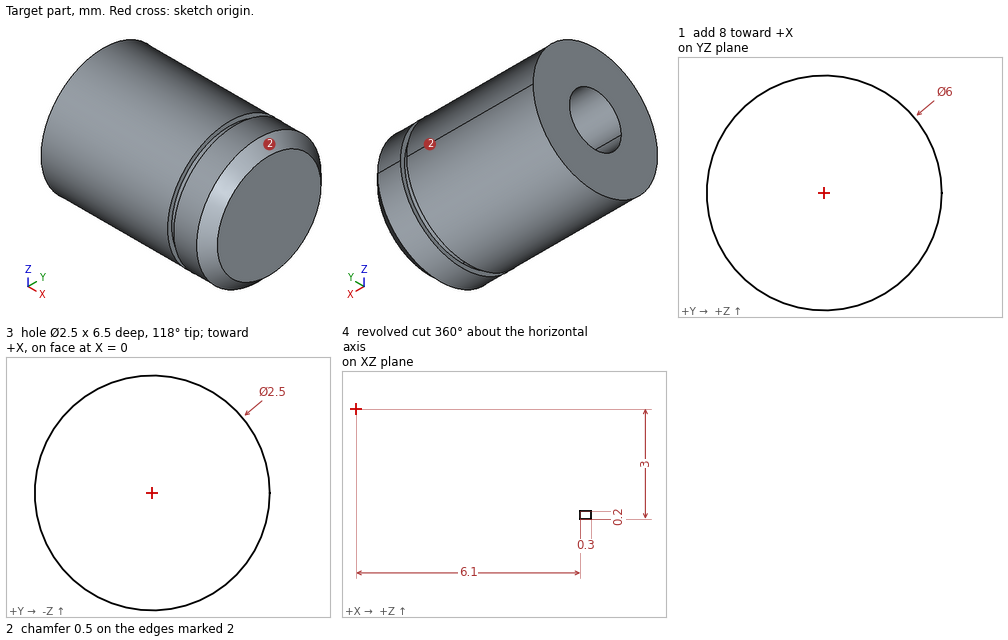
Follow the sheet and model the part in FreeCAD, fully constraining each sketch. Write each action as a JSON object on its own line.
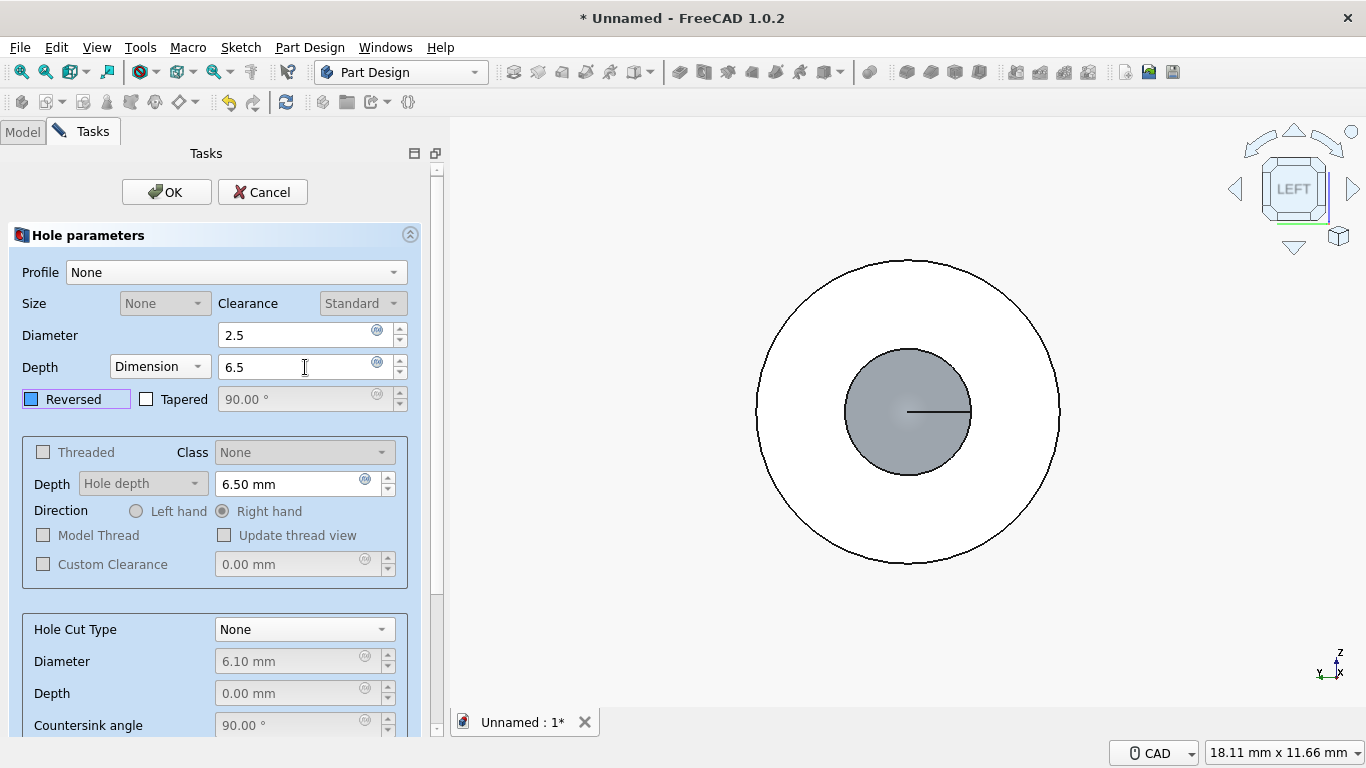
{"action": "left_click", "coordinate": [167, 192]}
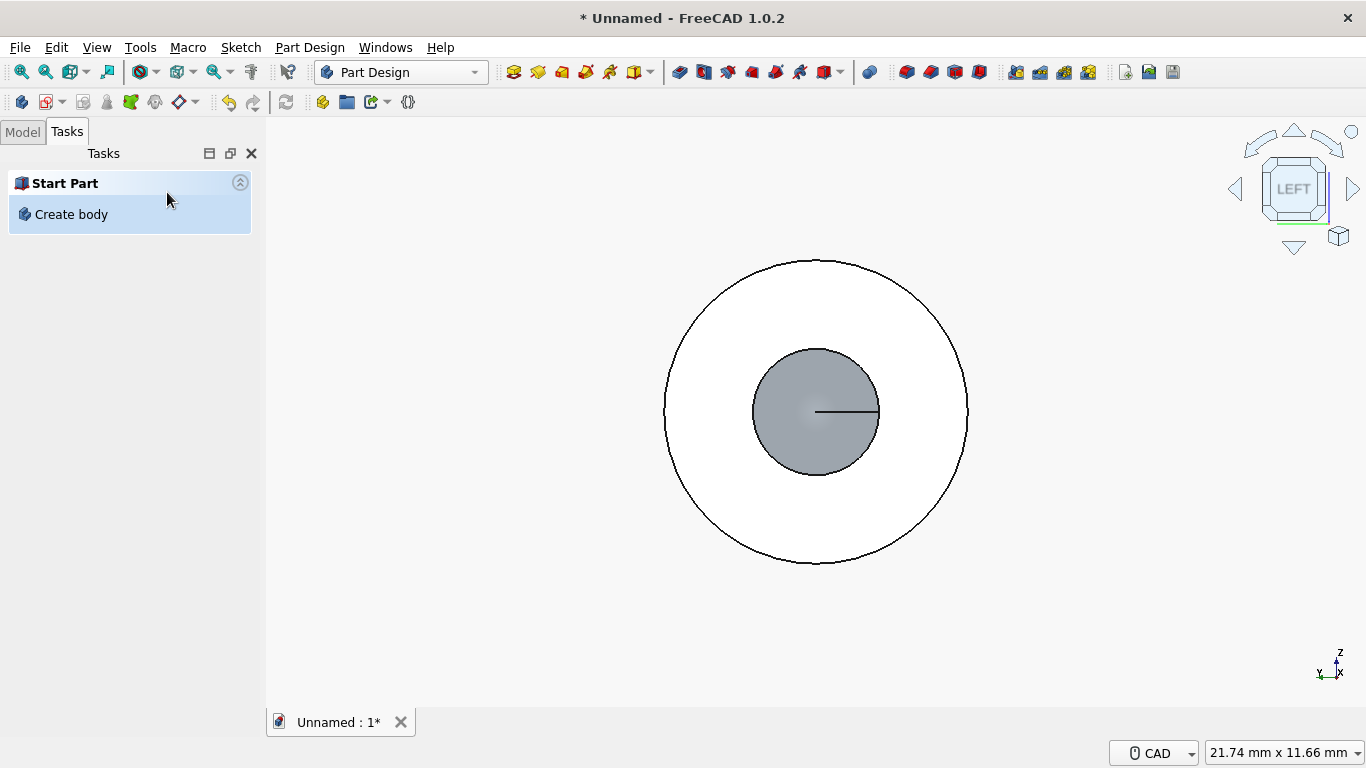
{"action": "left_click", "coordinate": [46, 102]}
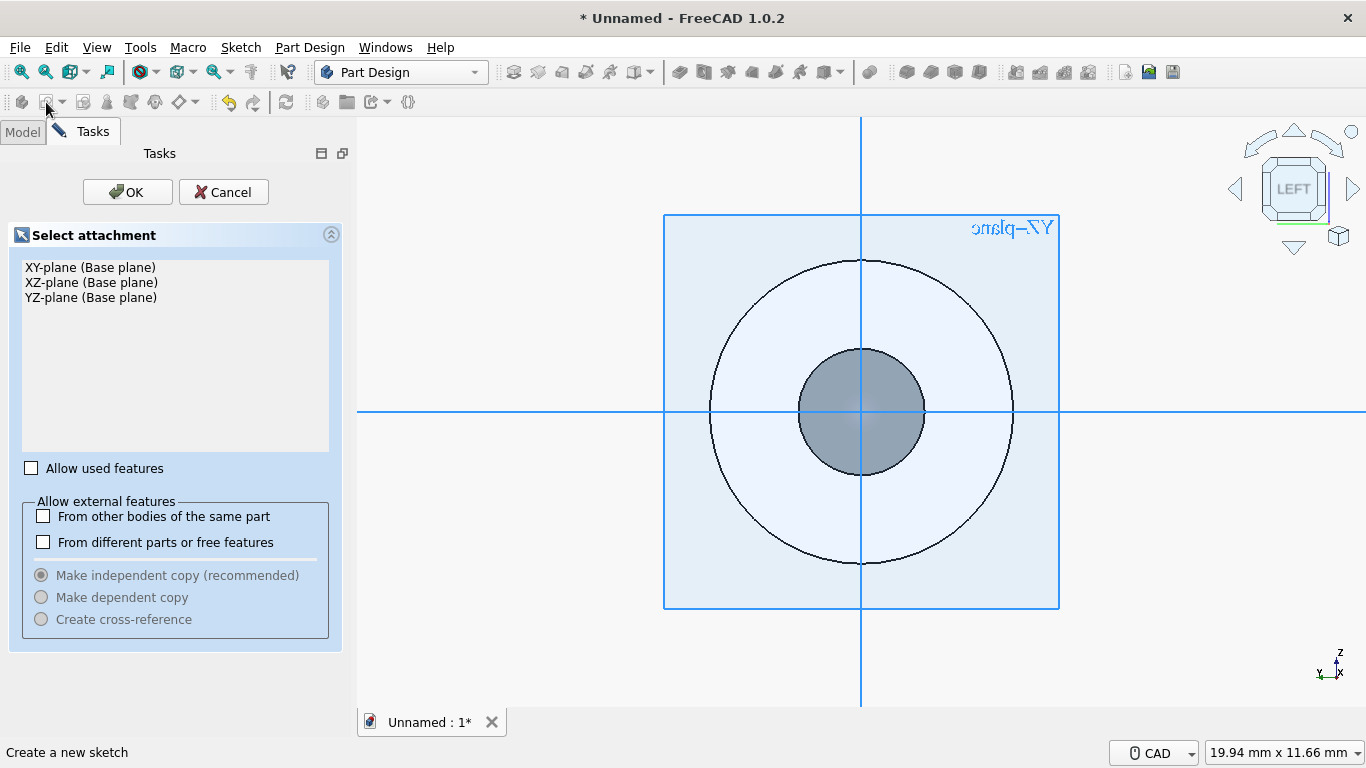
{"action": "left_click", "coordinate": [82, 282]}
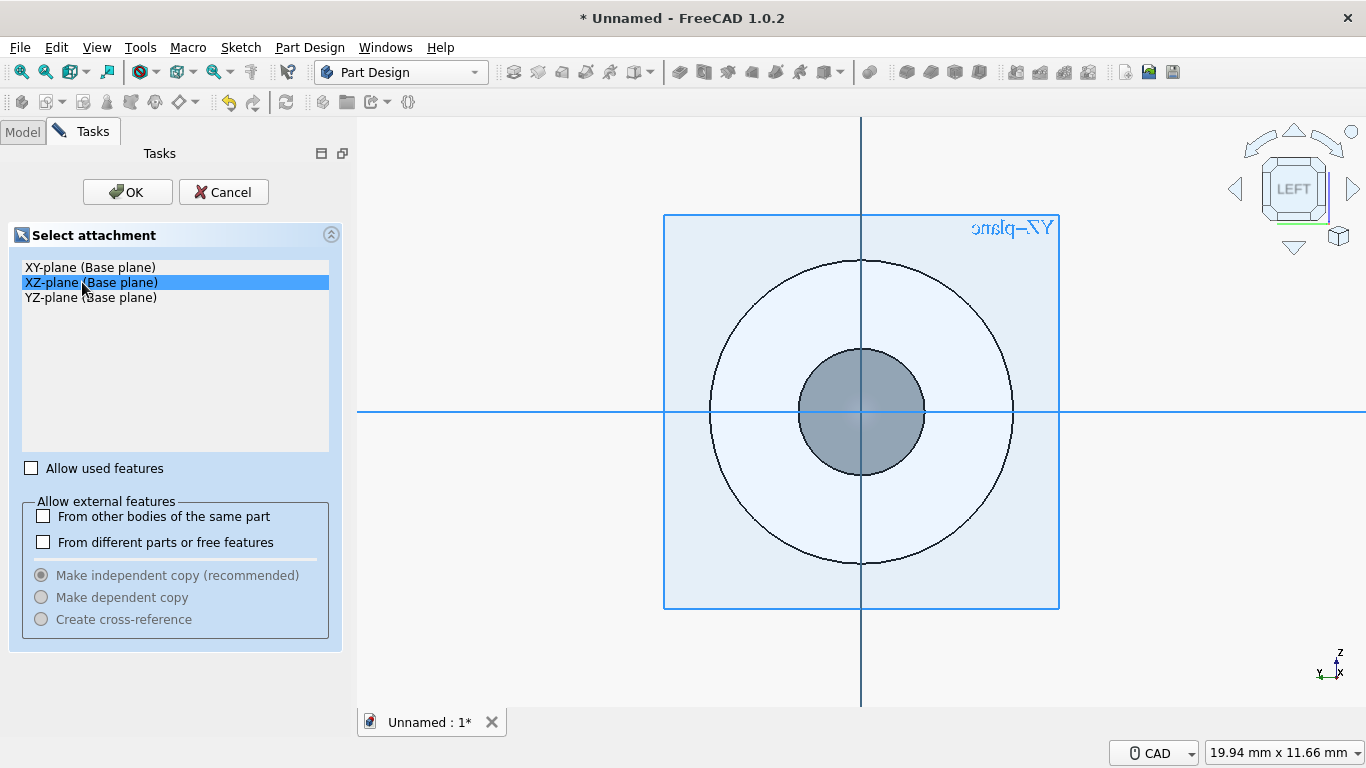
{"action": "left_click", "coordinate": [128, 192]}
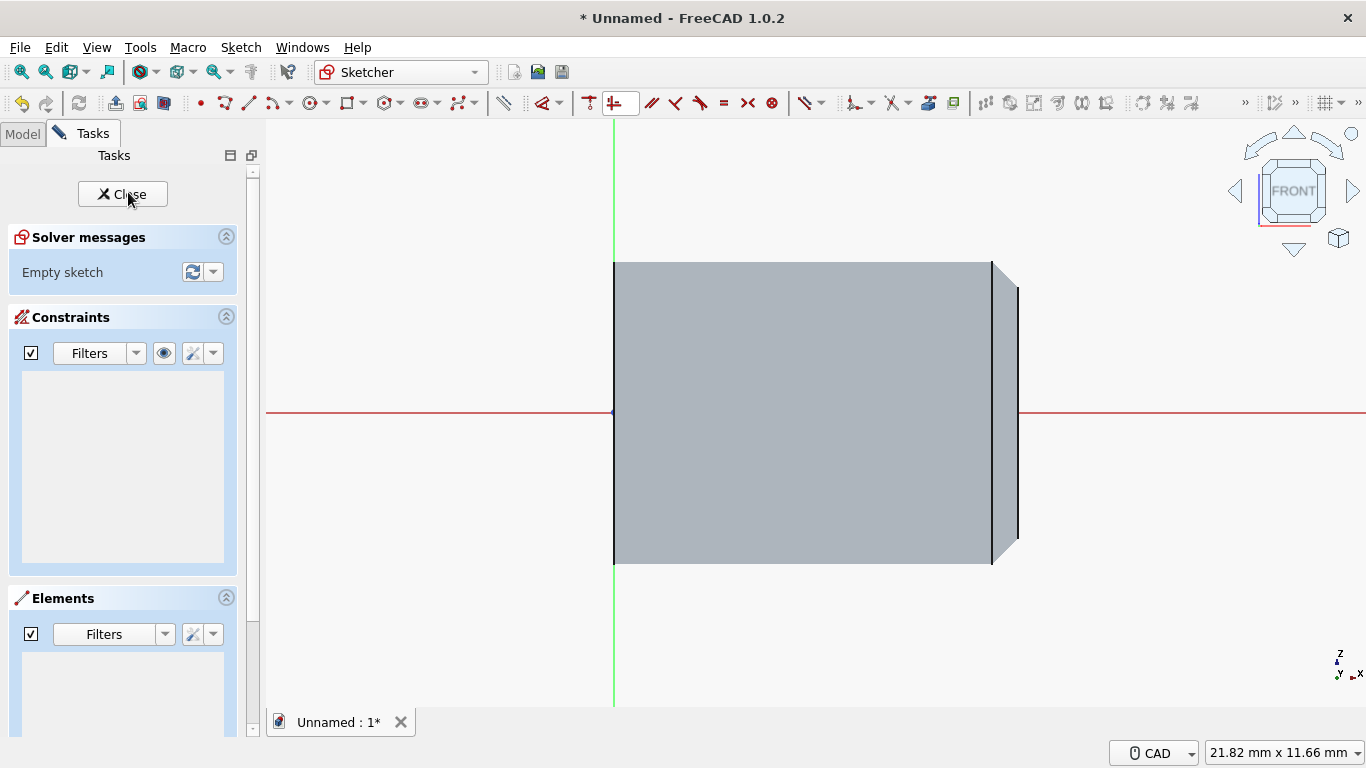
{"action": "left_click", "coordinate": [164, 104]}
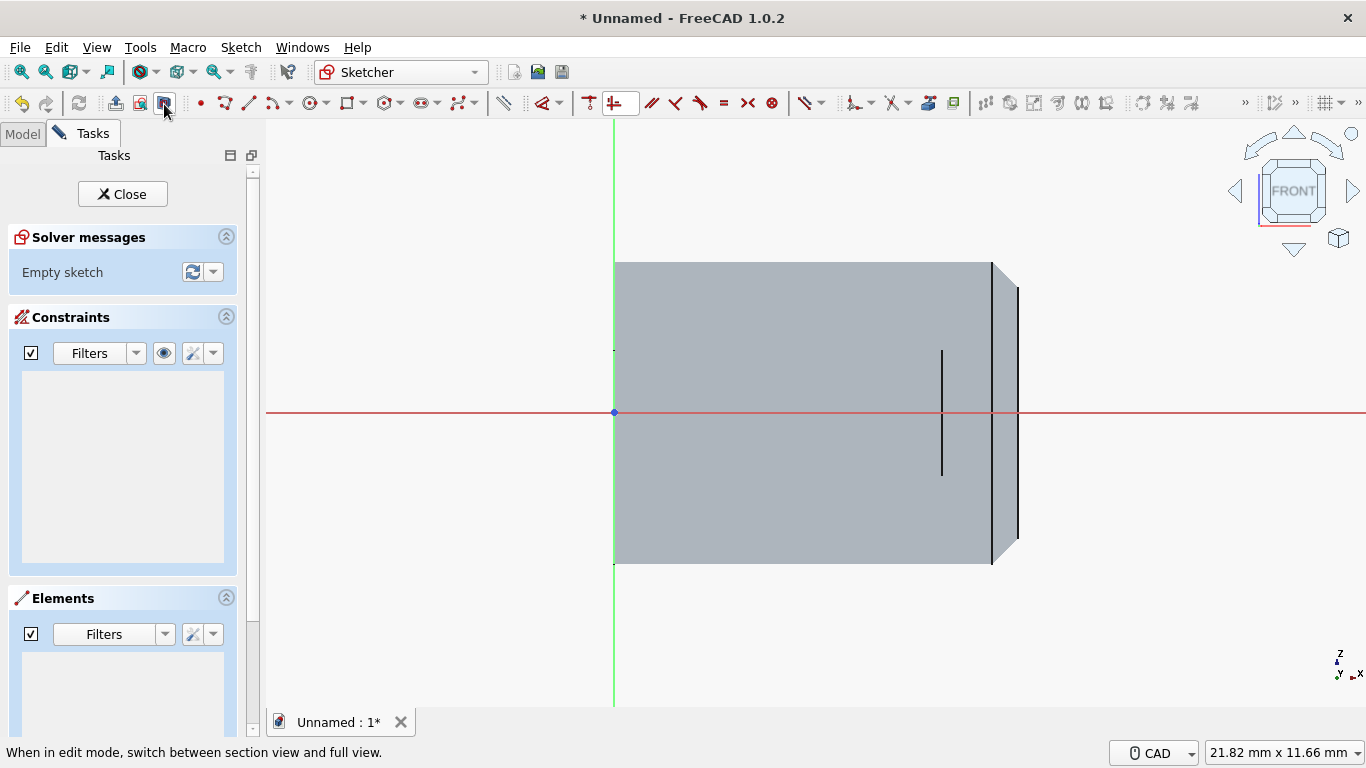
{"action": "scroll", "coordinate": [939, 567], "scroll_direction": "up", "scroll_amount": 15}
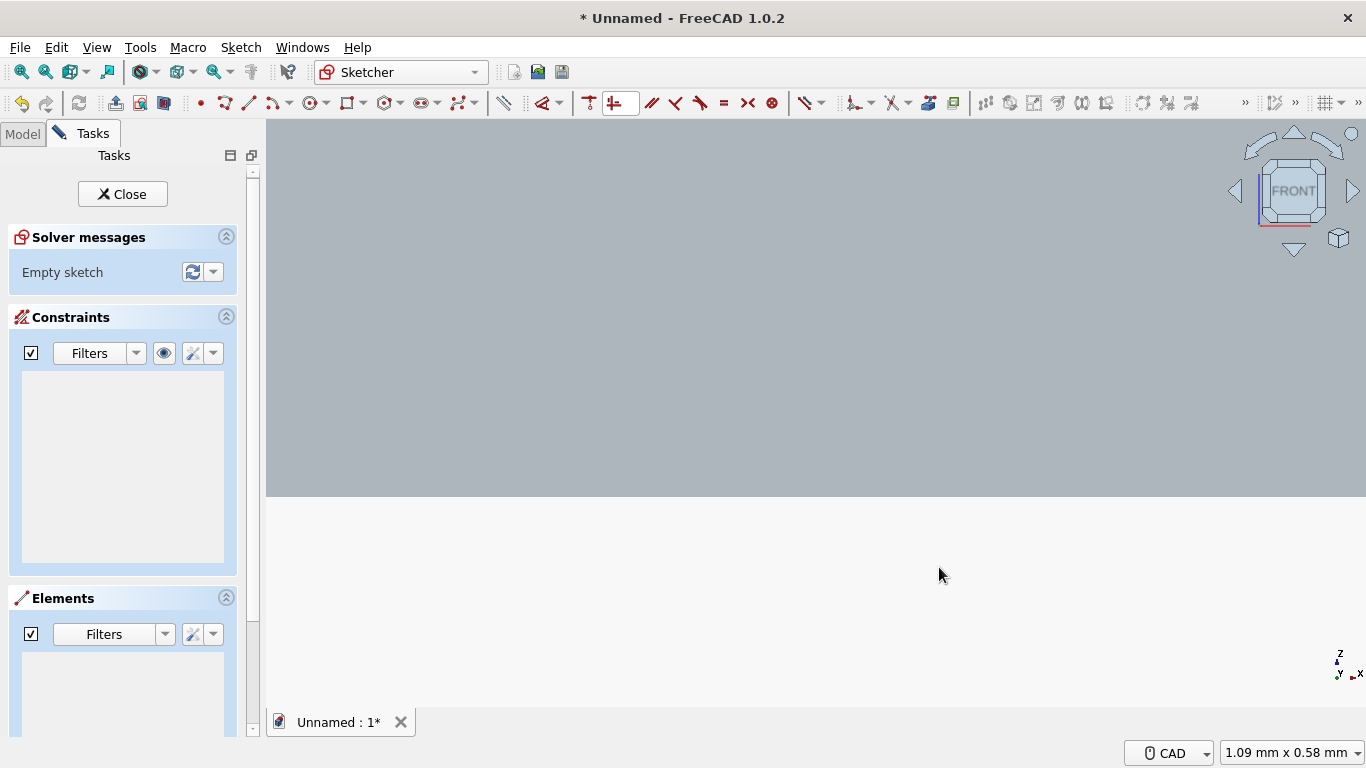
{"action": "scroll", "coordinate": [721, 376], "scroll_direction": "up", "scroll_amount": 3}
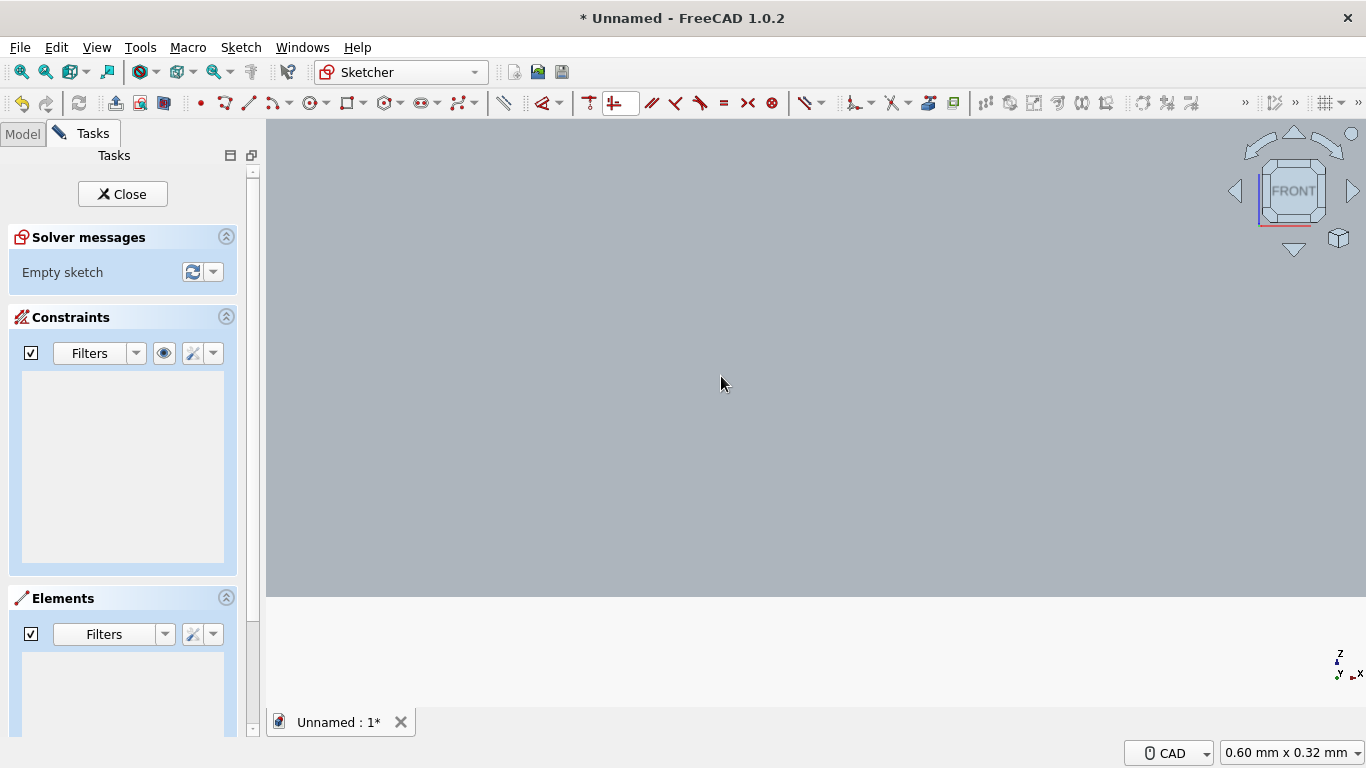
{"action": "key", "text": "g r"}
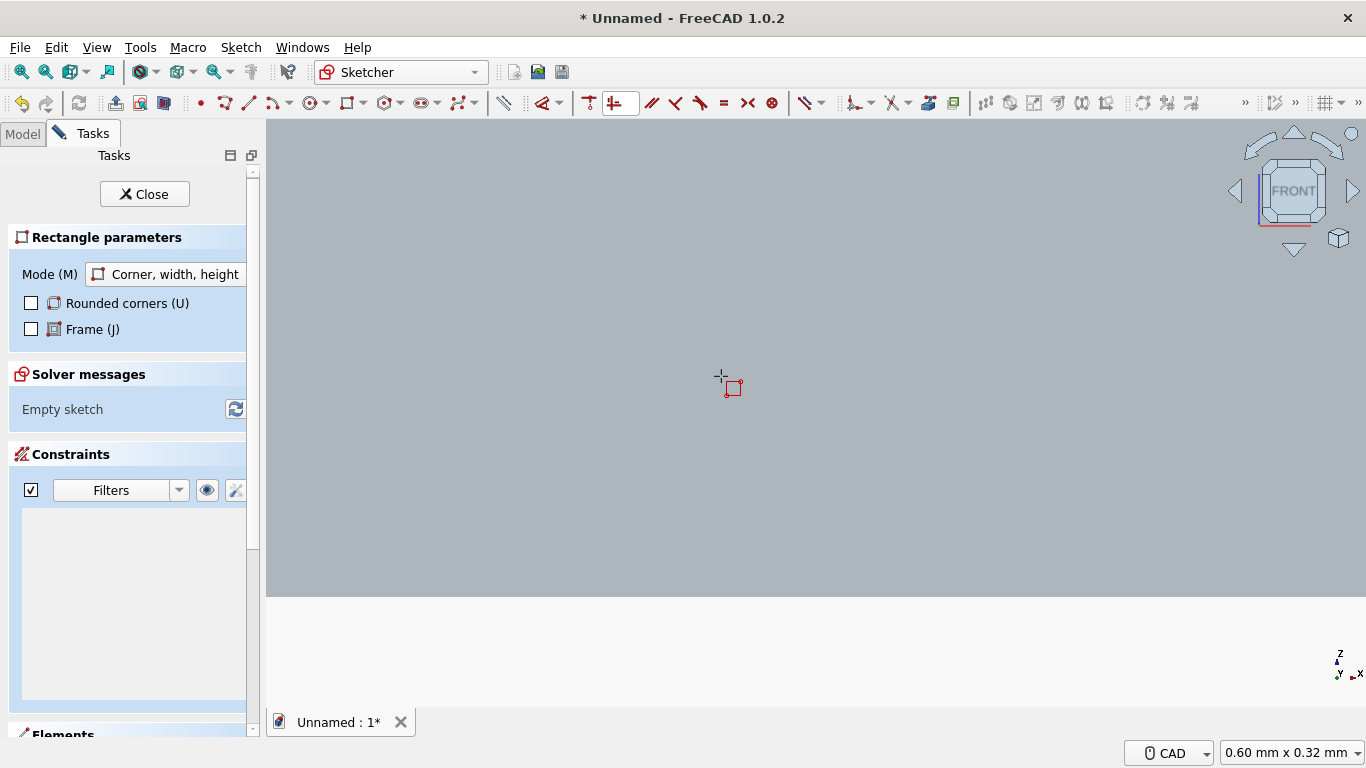
{"action": "left_click", "coordinate": [470, 228]}
{"action": "left_click", "coordinate": [1024, 597]}
{"action": "key", "text": "Escape"}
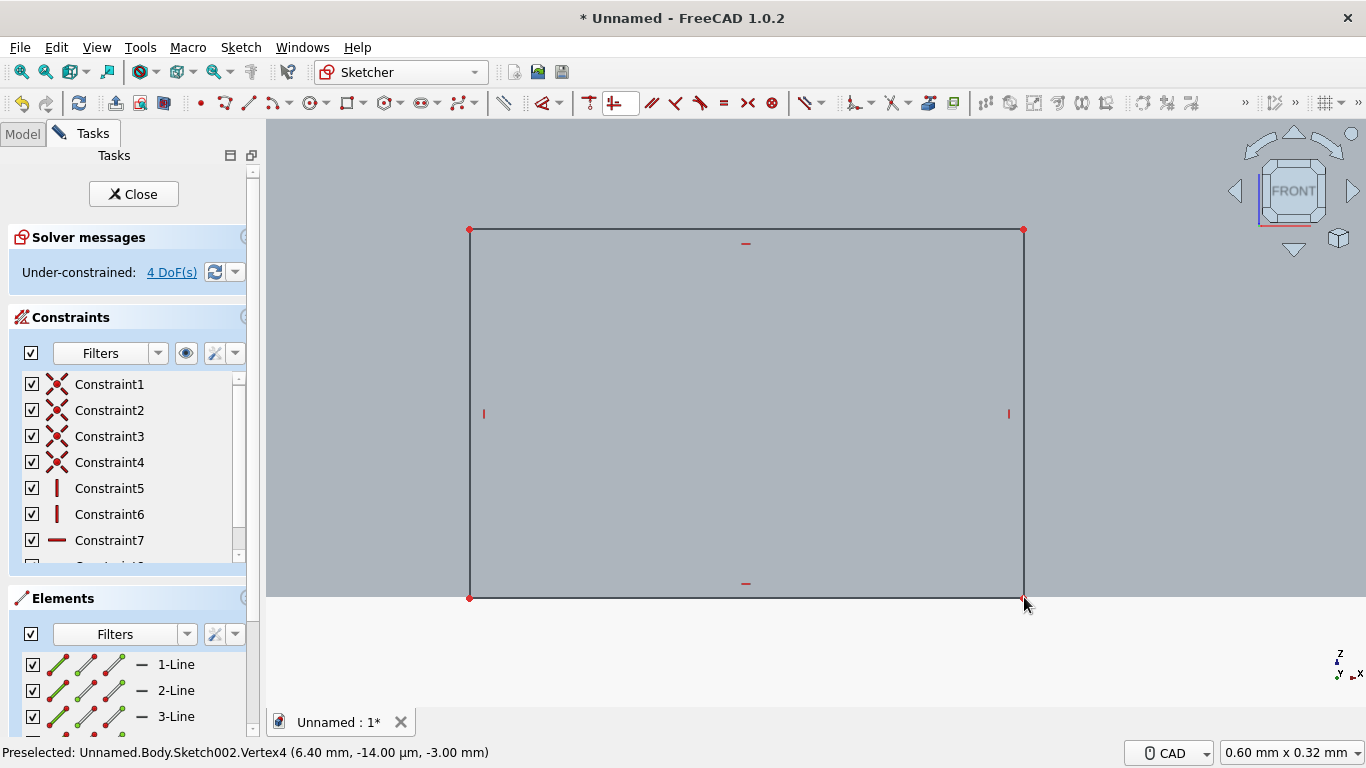
{"action": "key", "text": "d"}